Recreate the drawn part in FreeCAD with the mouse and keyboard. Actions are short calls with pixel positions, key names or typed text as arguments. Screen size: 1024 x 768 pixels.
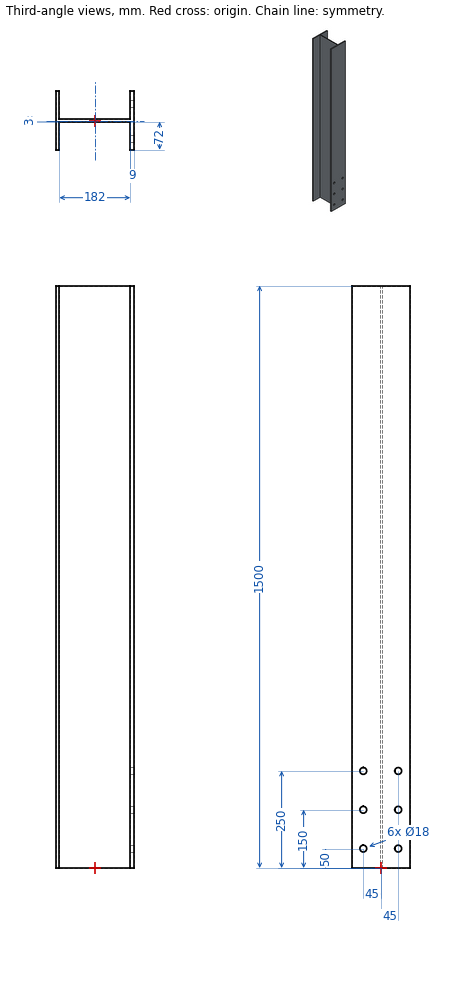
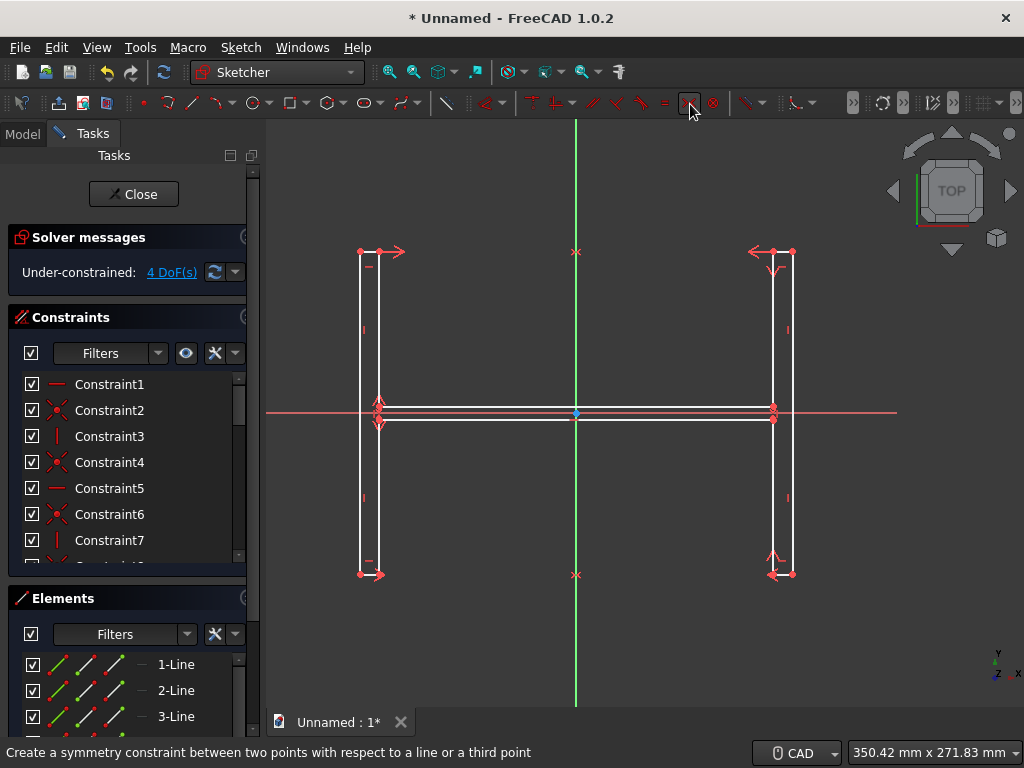
click(486, 104)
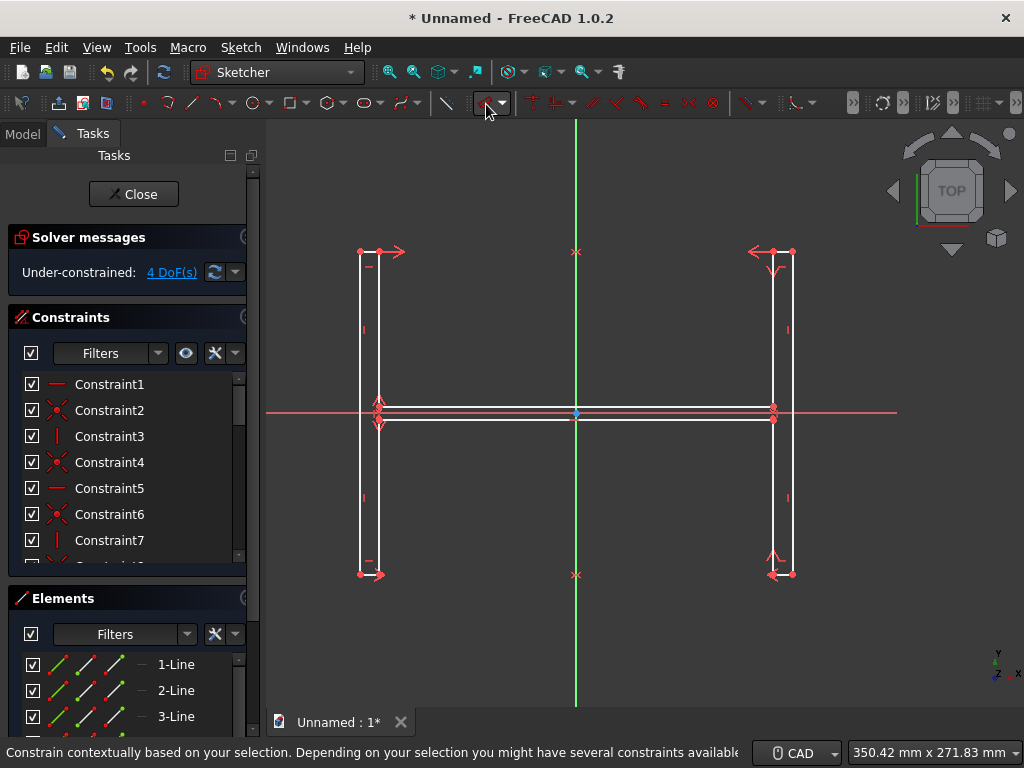
scroll(783, 575, up, 4)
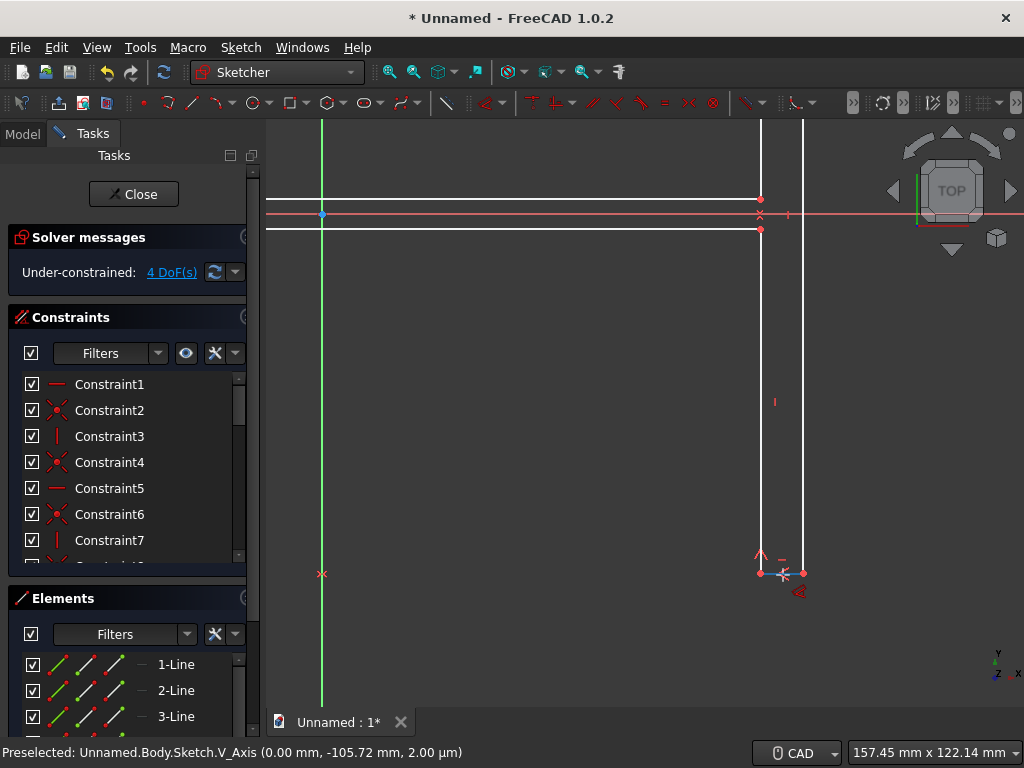
click(782, 574)
click(782, 608)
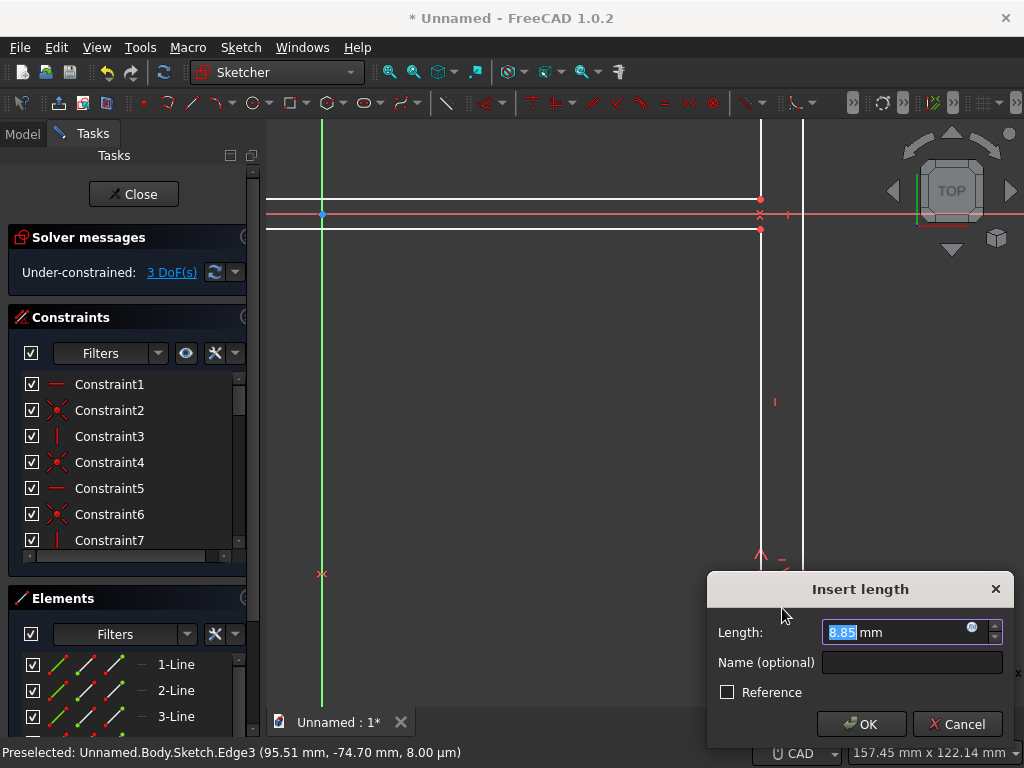
text(9)
key(Return)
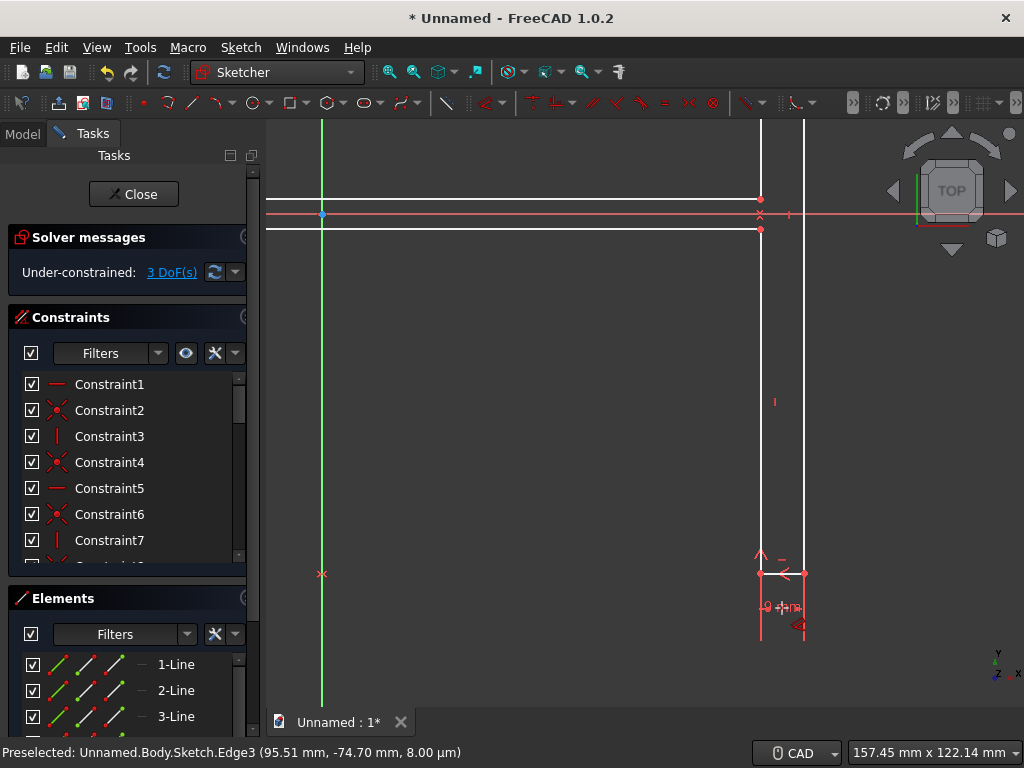
click(761, 333)
click(727, 402)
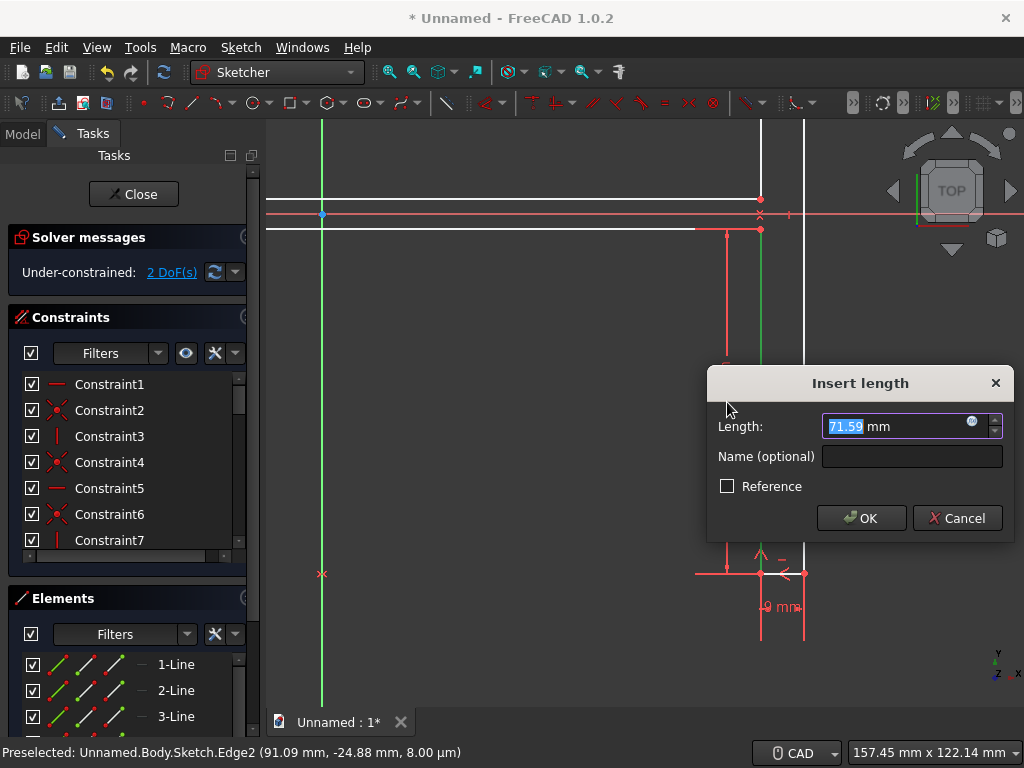
text(72)
key(Return)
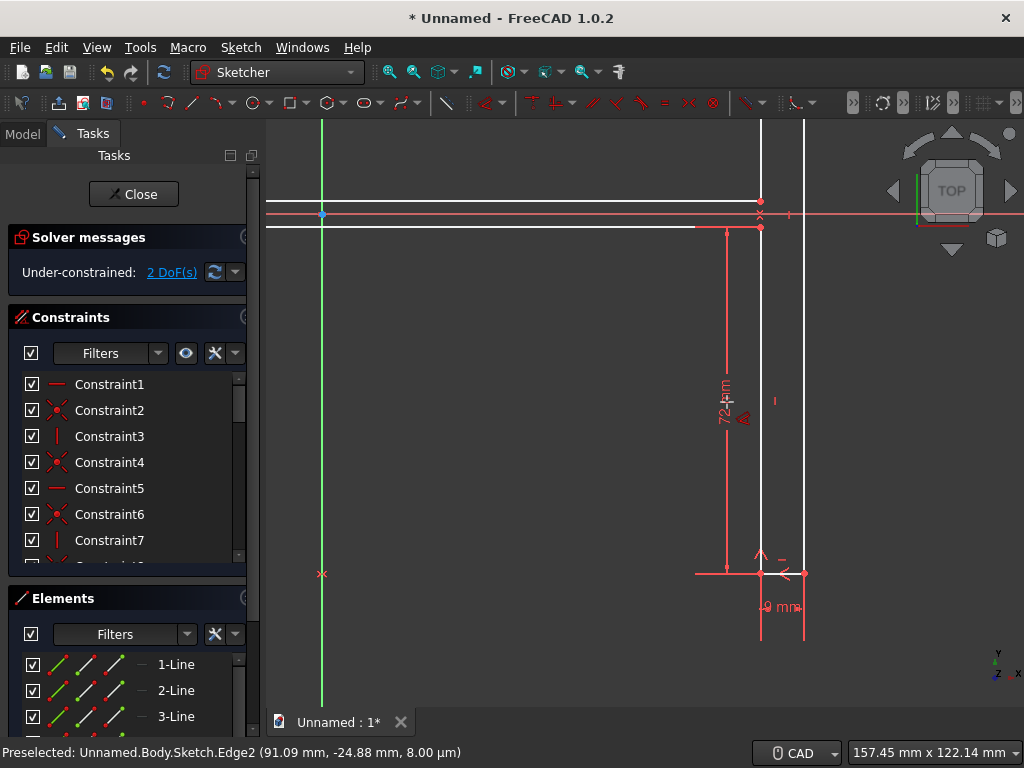
scroll(784, 575, down, 4)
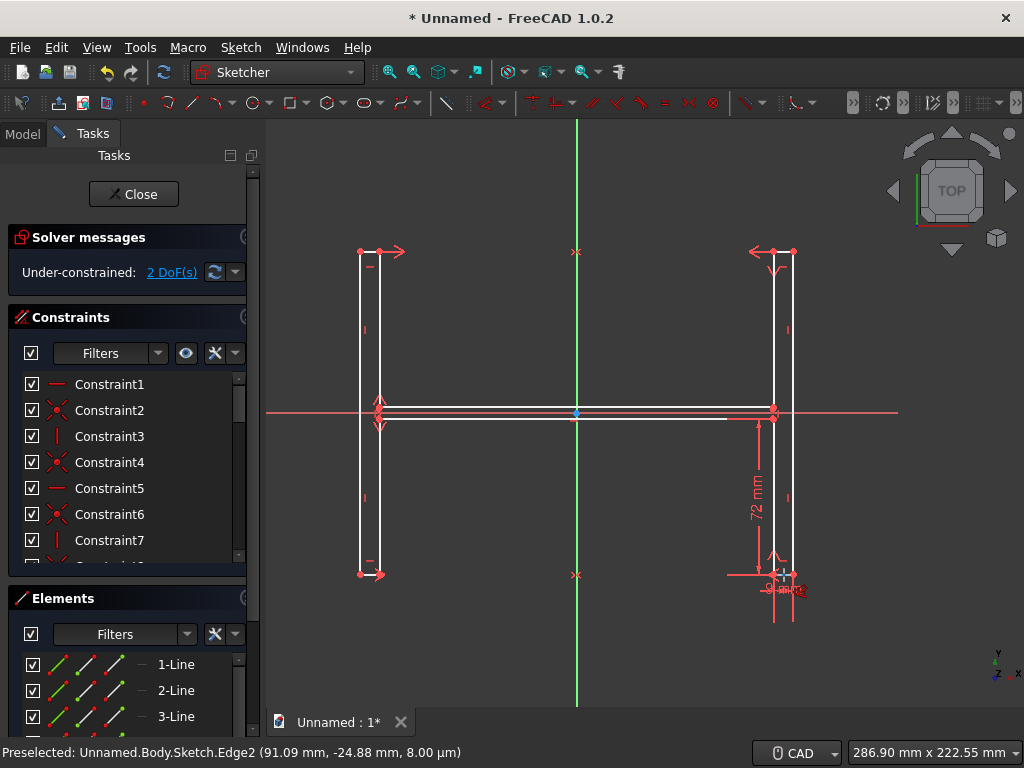
scroll(380, 419, up, 10)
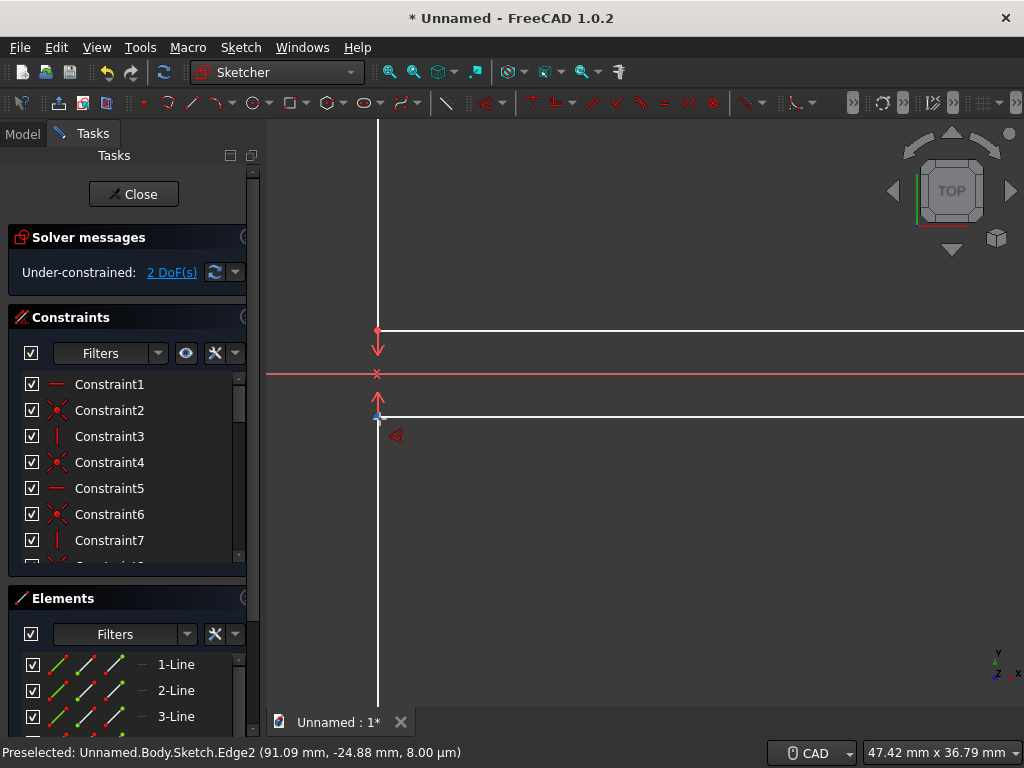
click(378, 417)
click(344, 395)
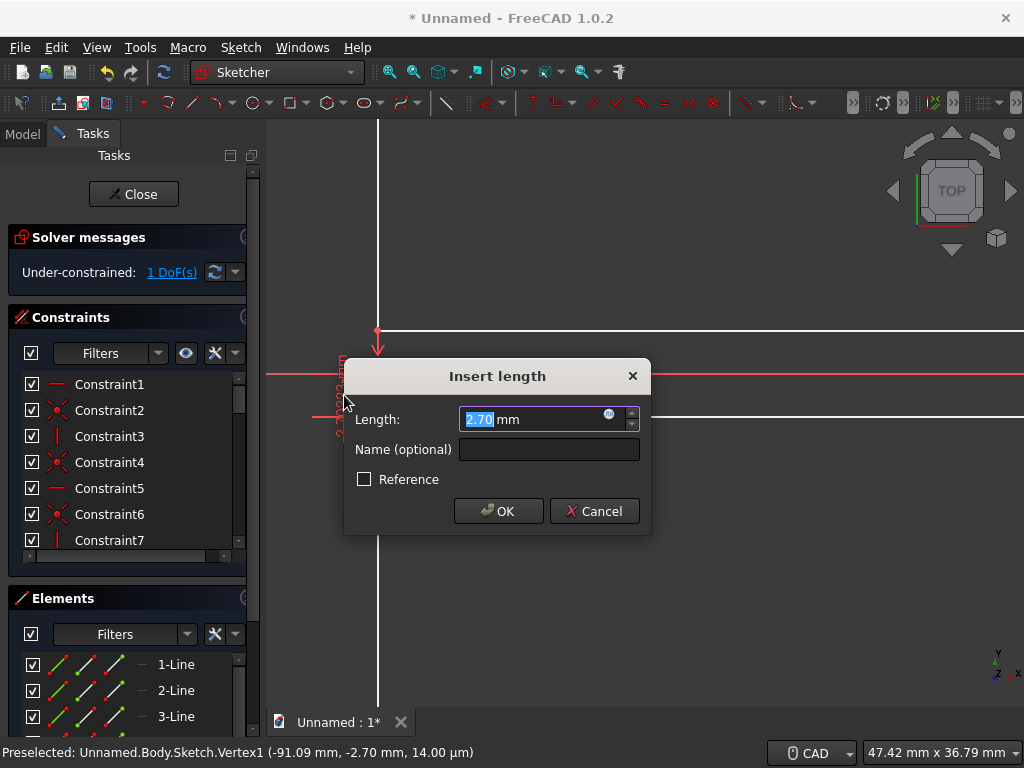
text(3)
key(Return)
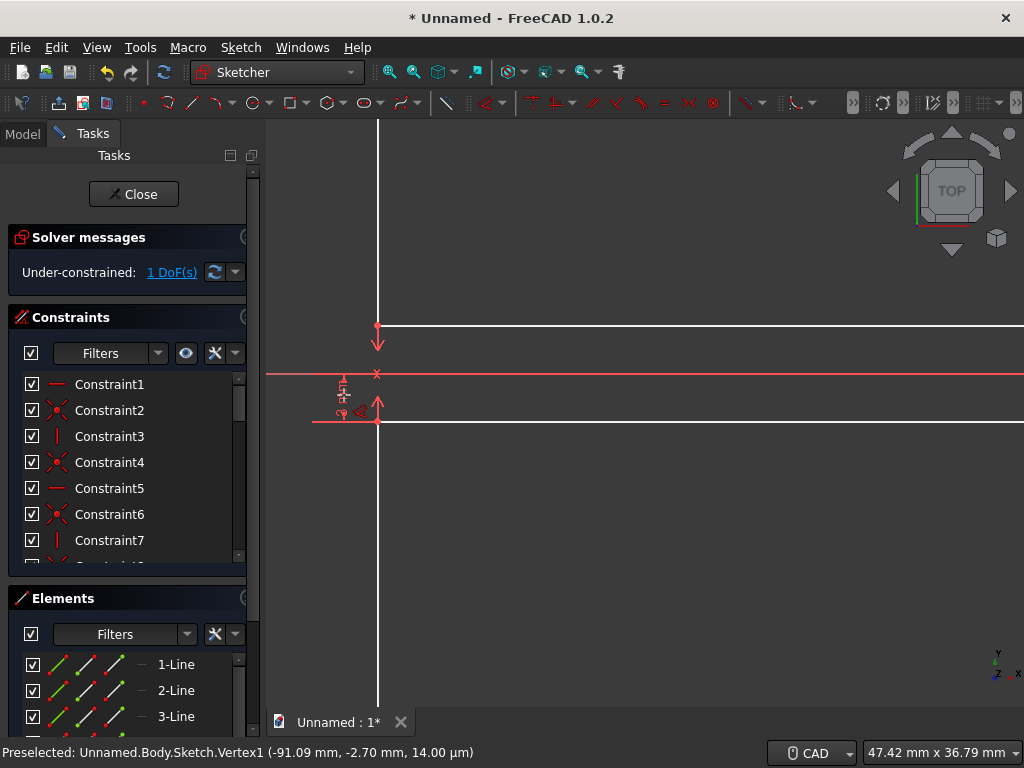
scroll(380, 419, down, 10)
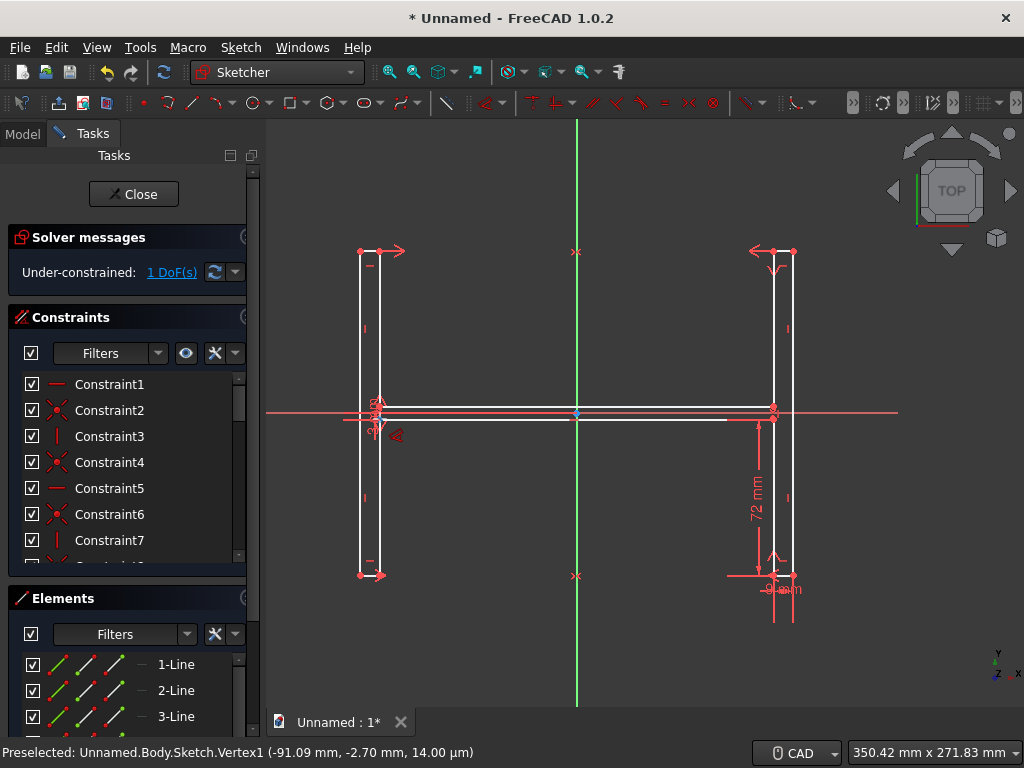
scroll(498, 420, up, 4)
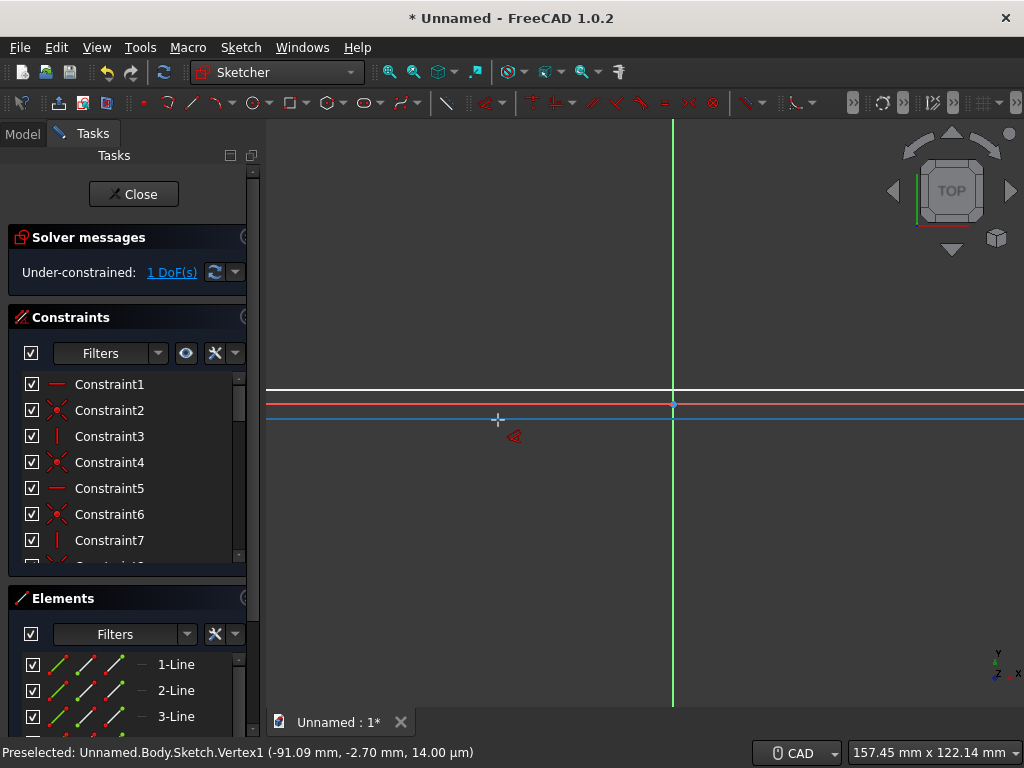
click(498, 419)
click(576, 453)